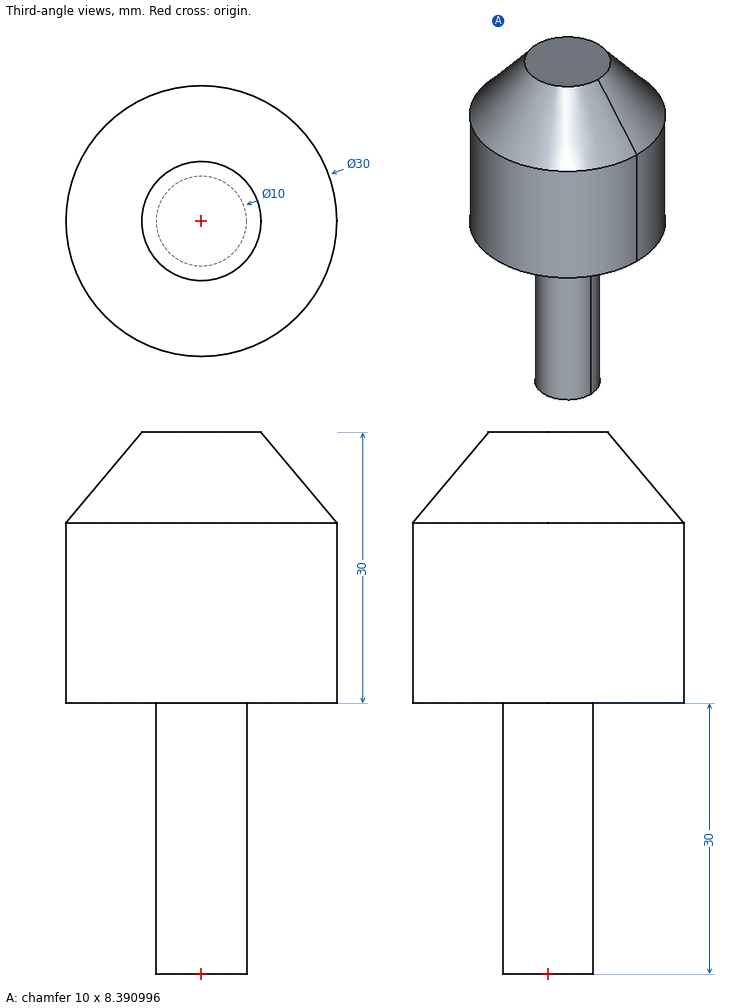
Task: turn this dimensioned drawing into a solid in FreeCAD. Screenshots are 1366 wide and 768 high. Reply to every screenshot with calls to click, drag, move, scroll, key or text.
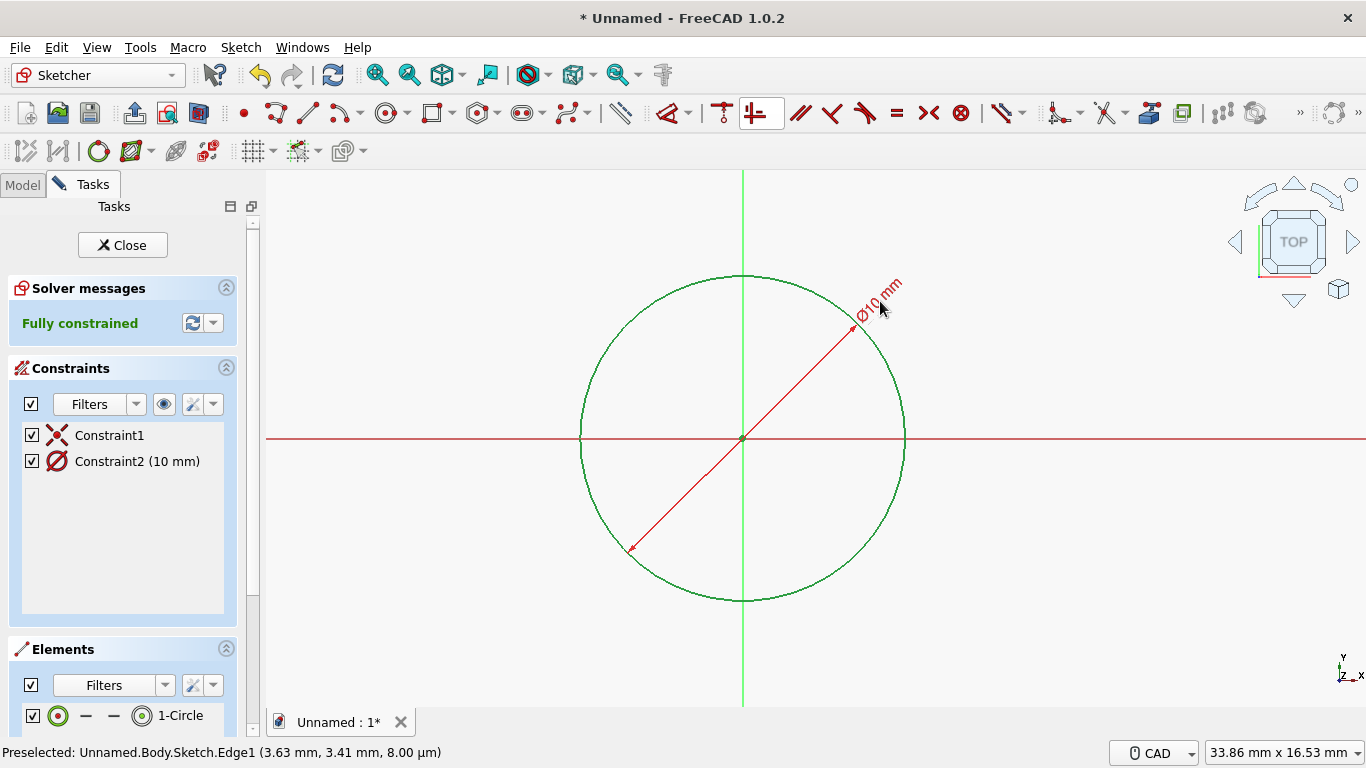
click(123, 245)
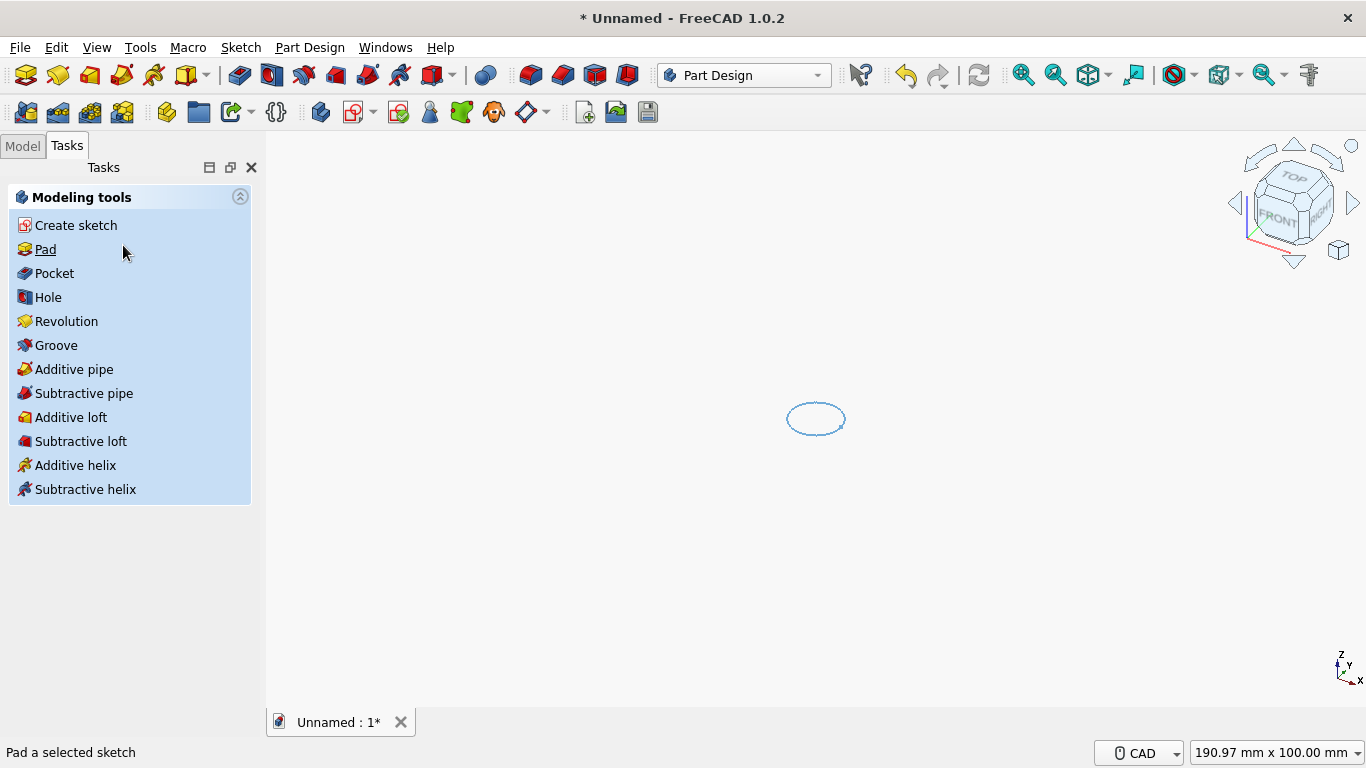
click(26, 76)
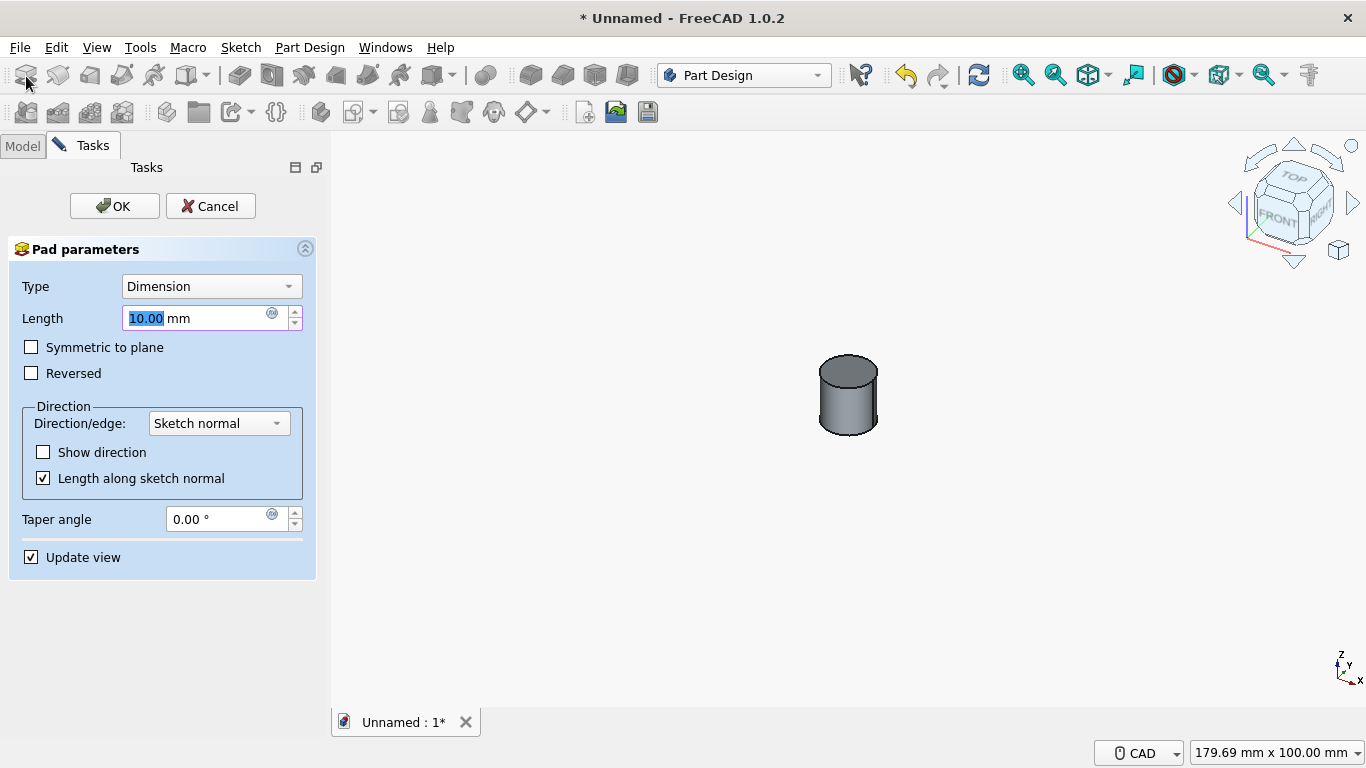
text(30)
key(Tab)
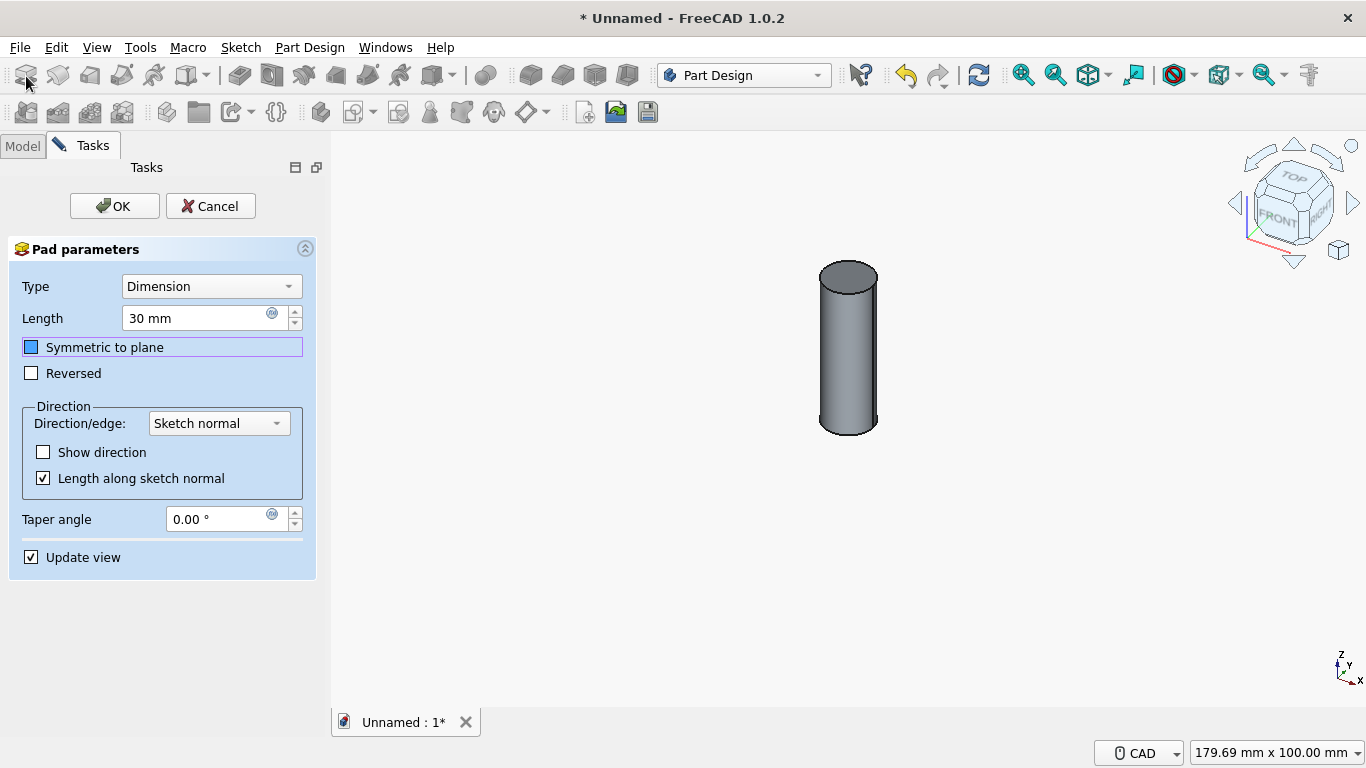
click(115, 206)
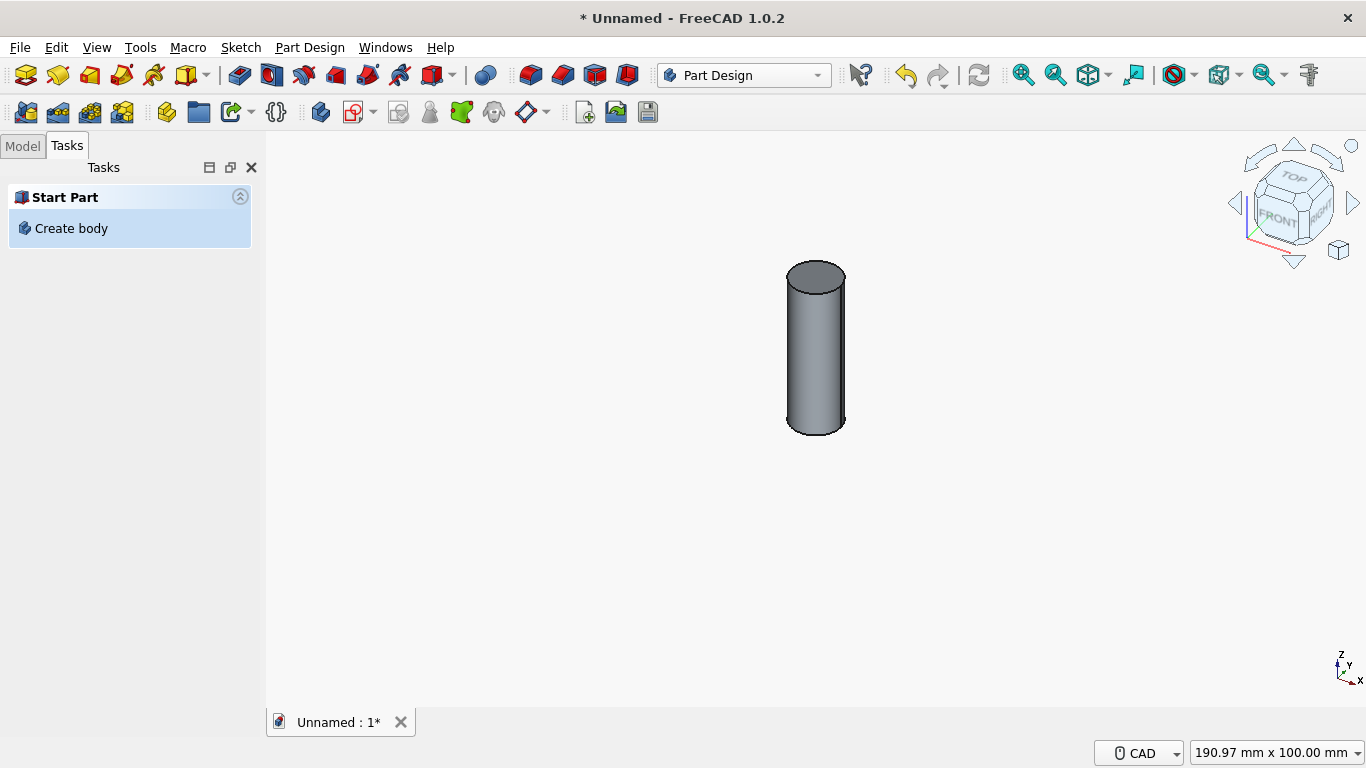
click(1024, 76)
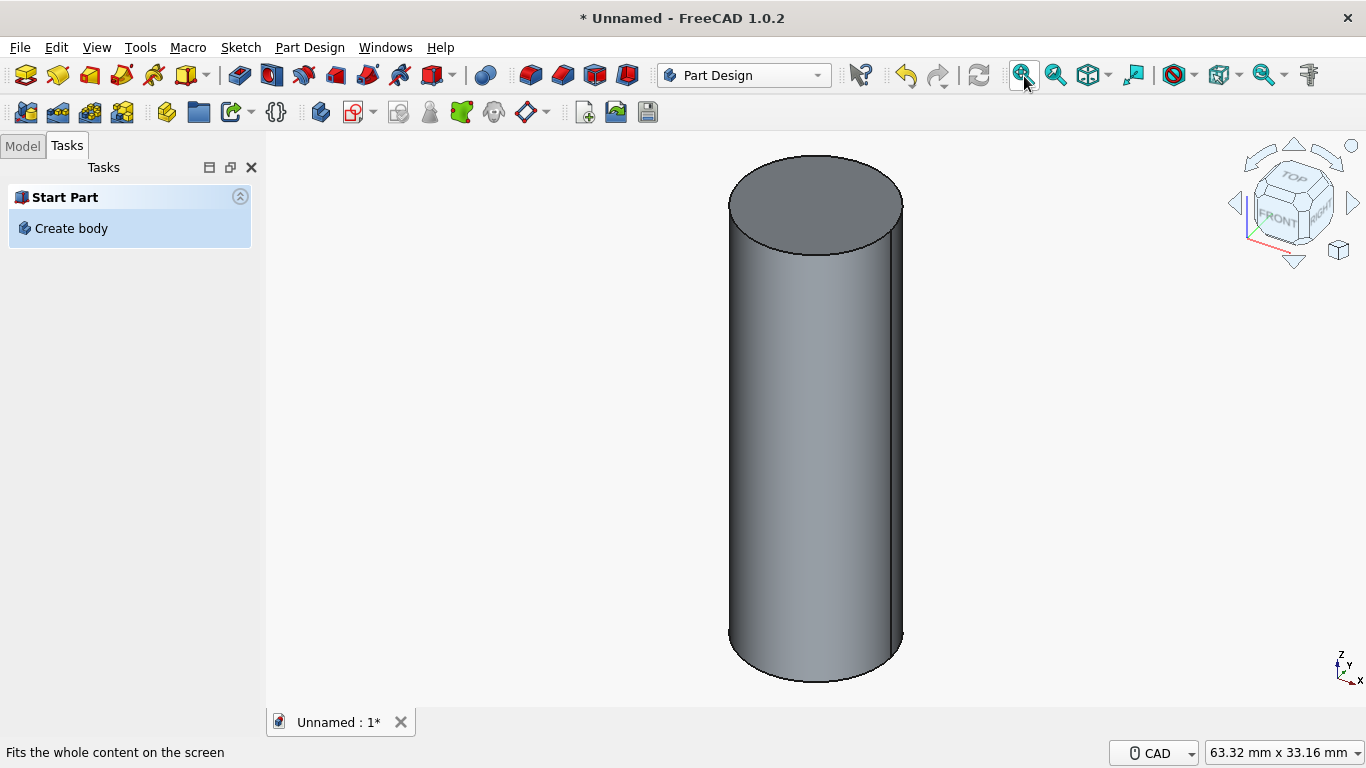
click(816, 205)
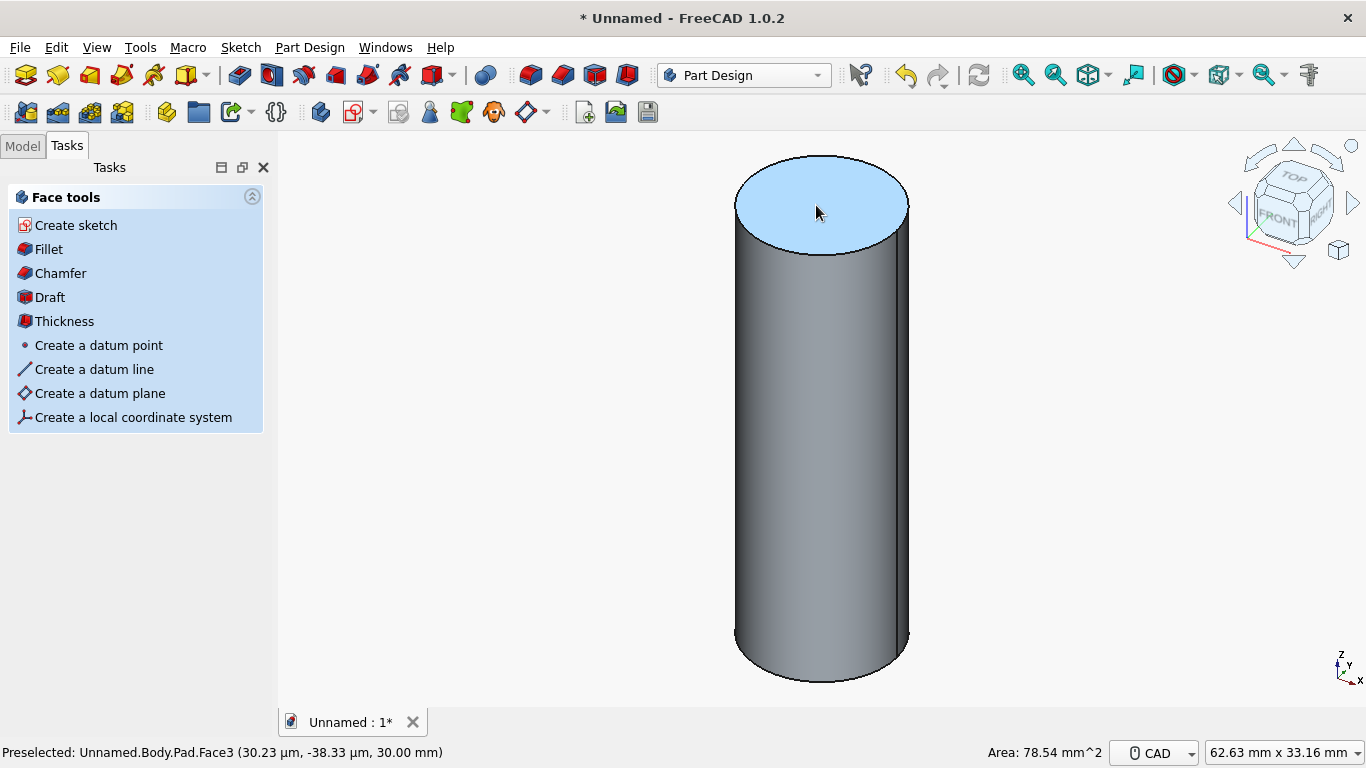
click(354, 112)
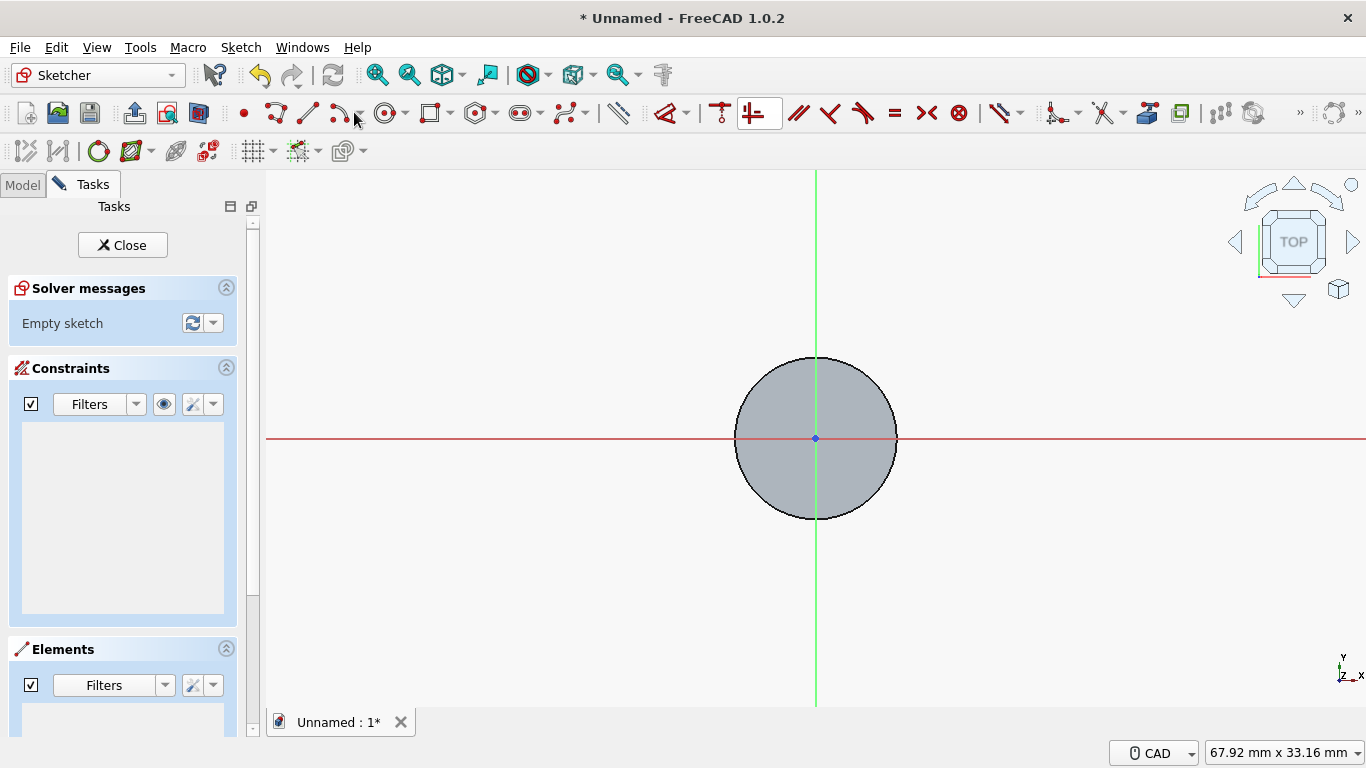
scroll(608, 438, down, 2)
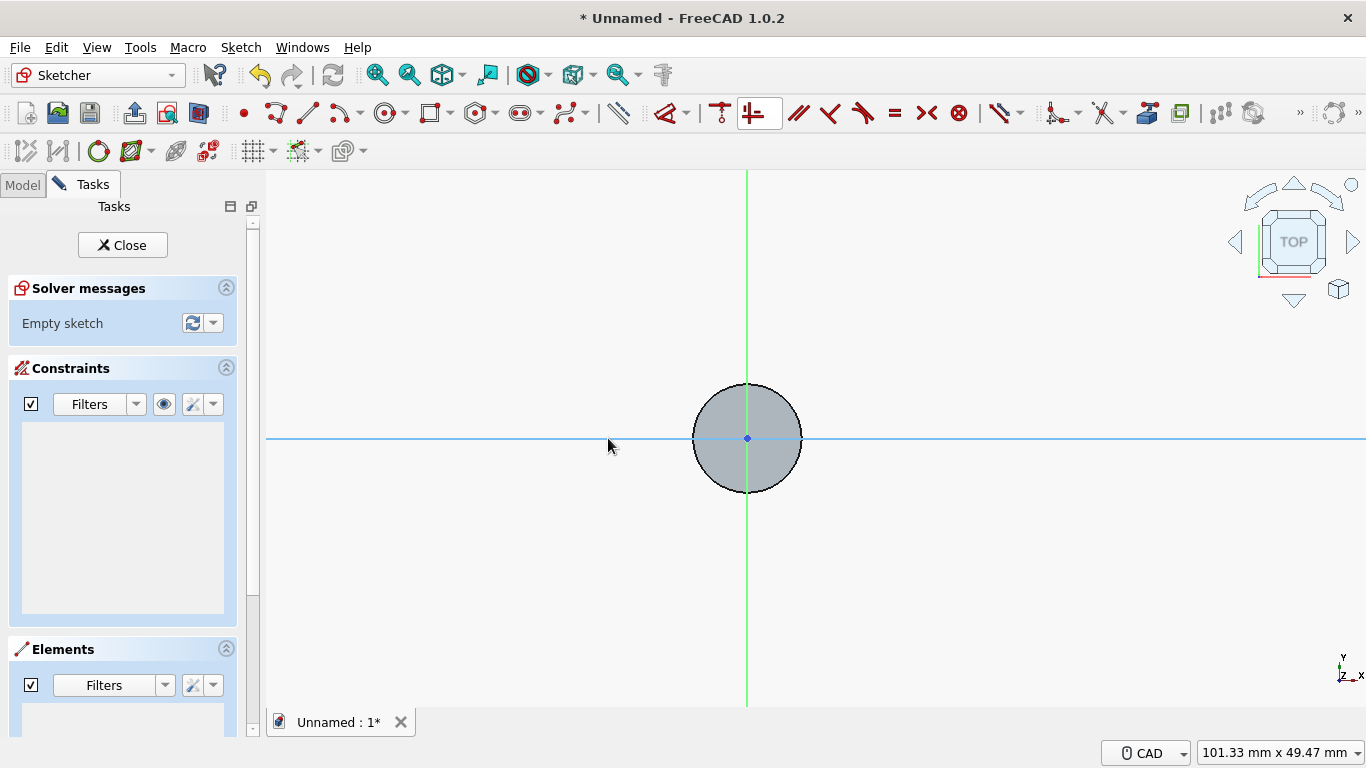
click(386, 114)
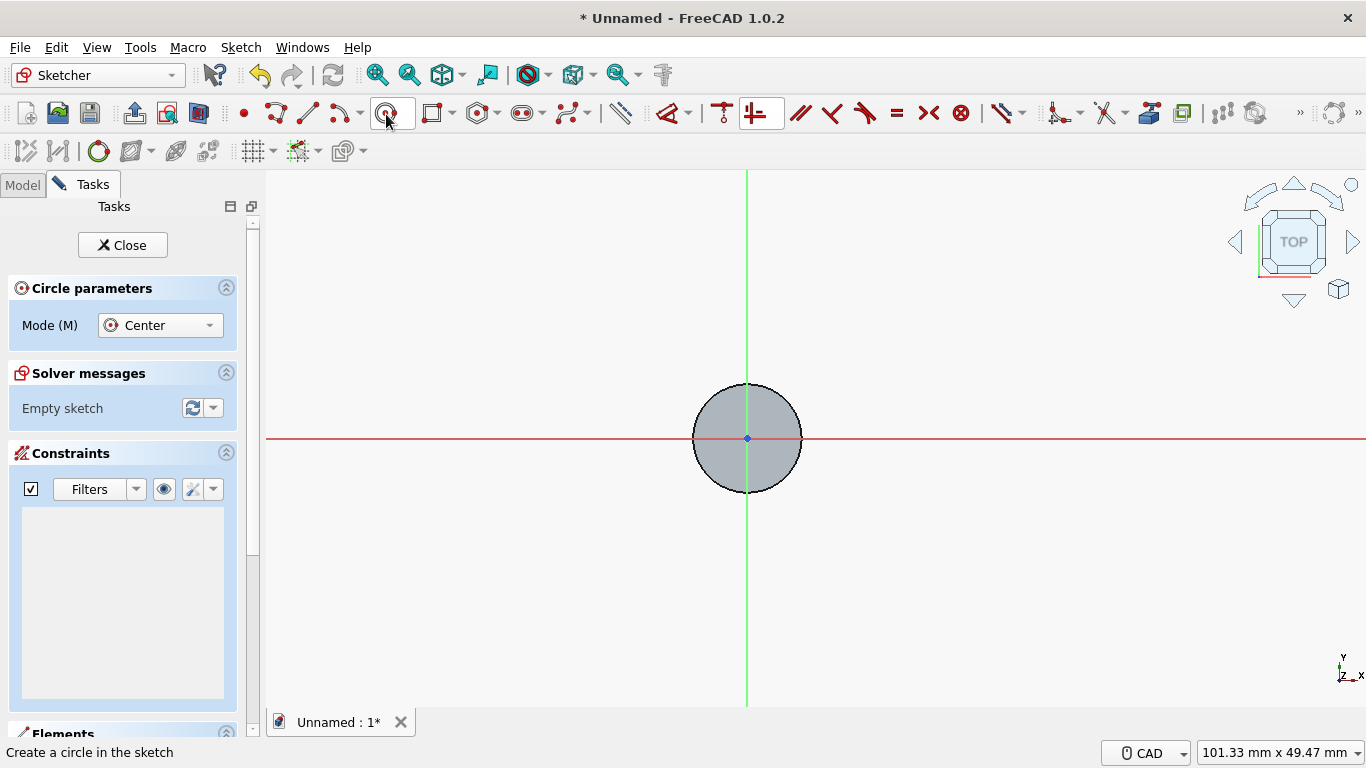
click(747, 438)
click(863, 323)
key(Escape)